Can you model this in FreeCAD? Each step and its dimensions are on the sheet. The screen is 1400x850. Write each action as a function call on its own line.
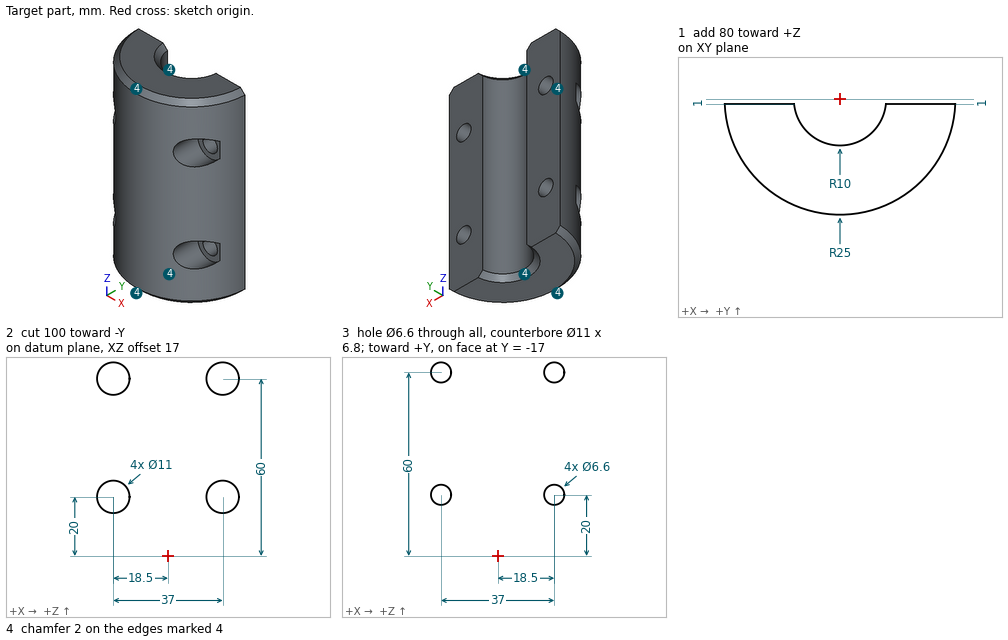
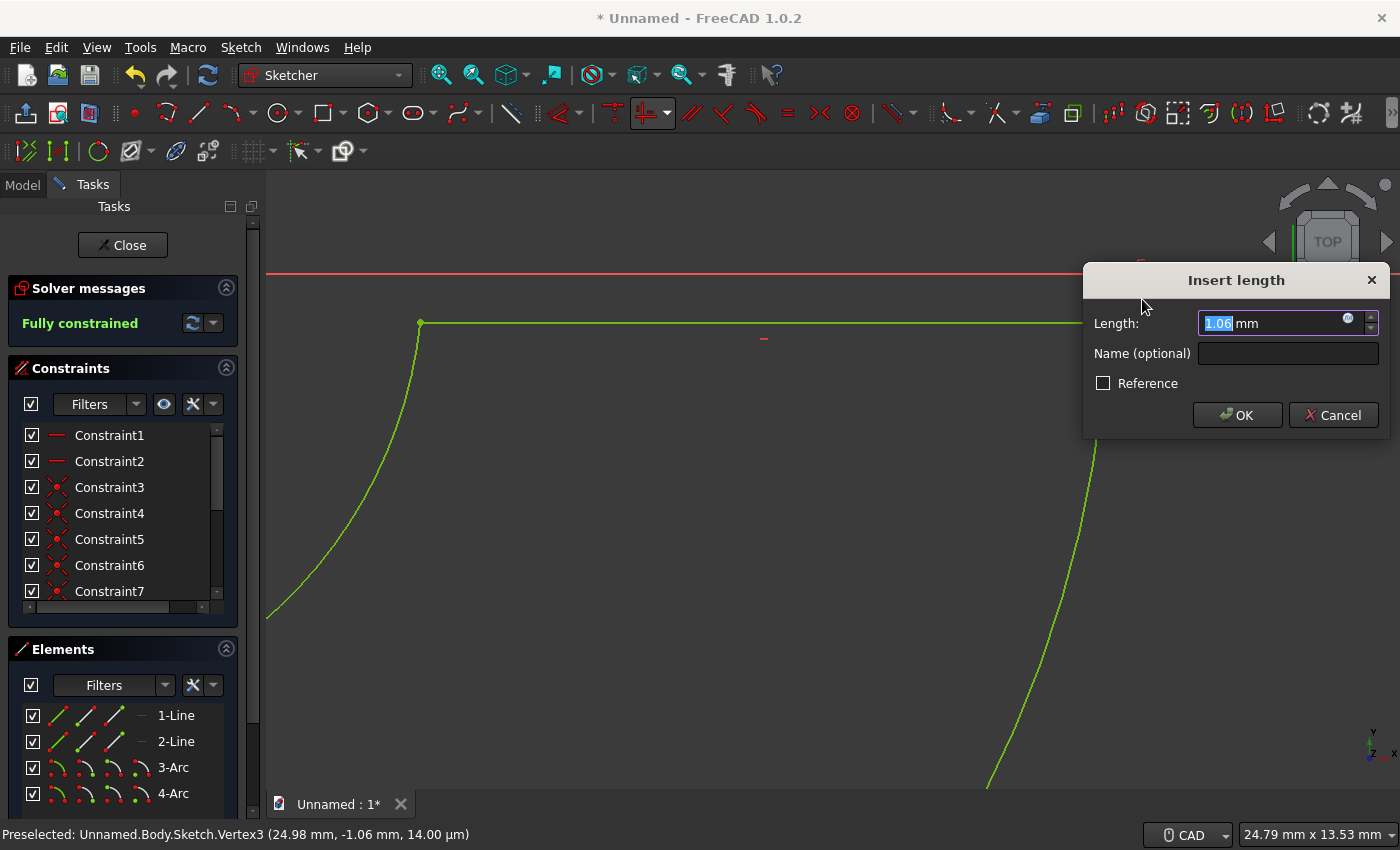
text(1)
key(Return)
key(Escape)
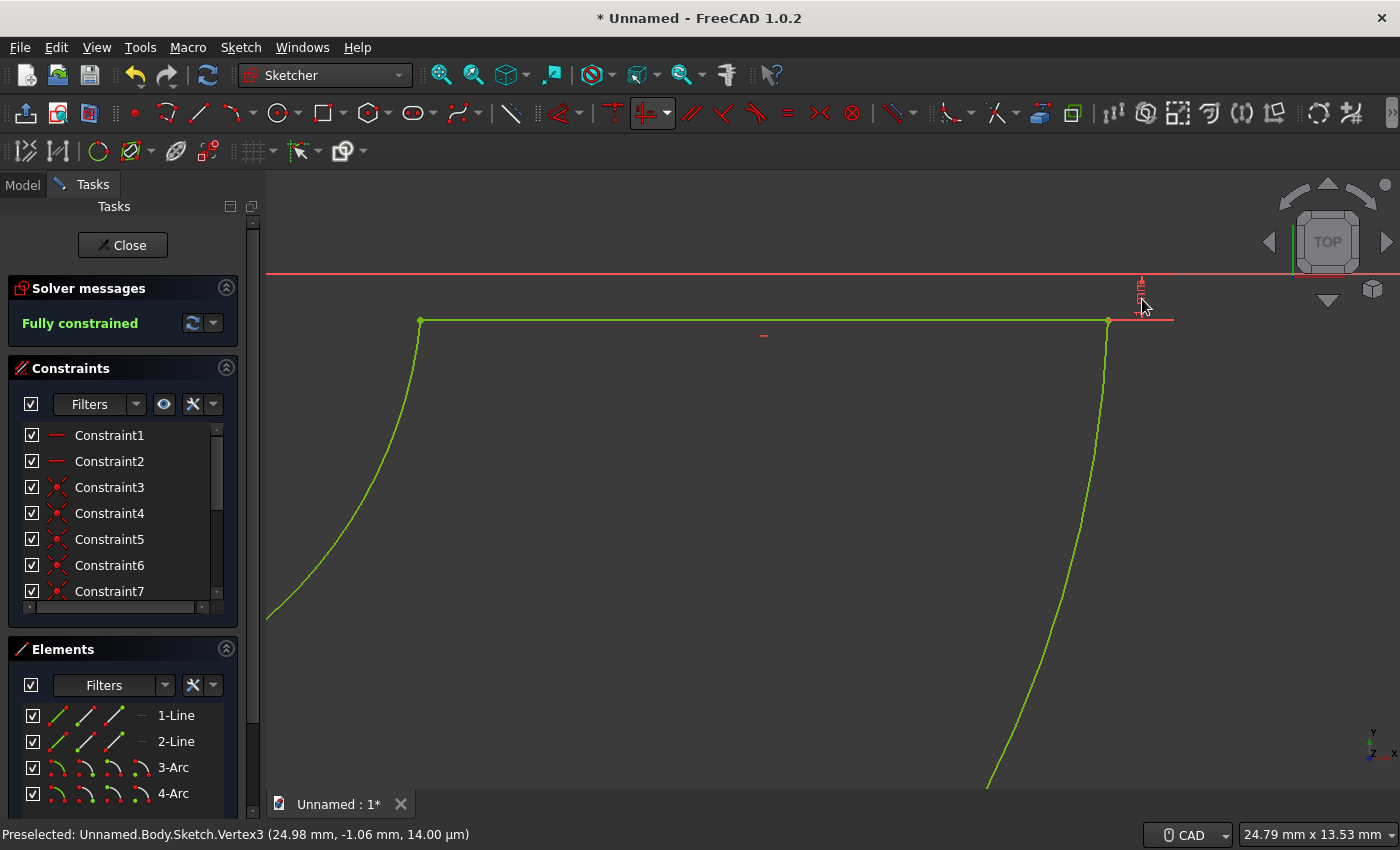
click(123, 245)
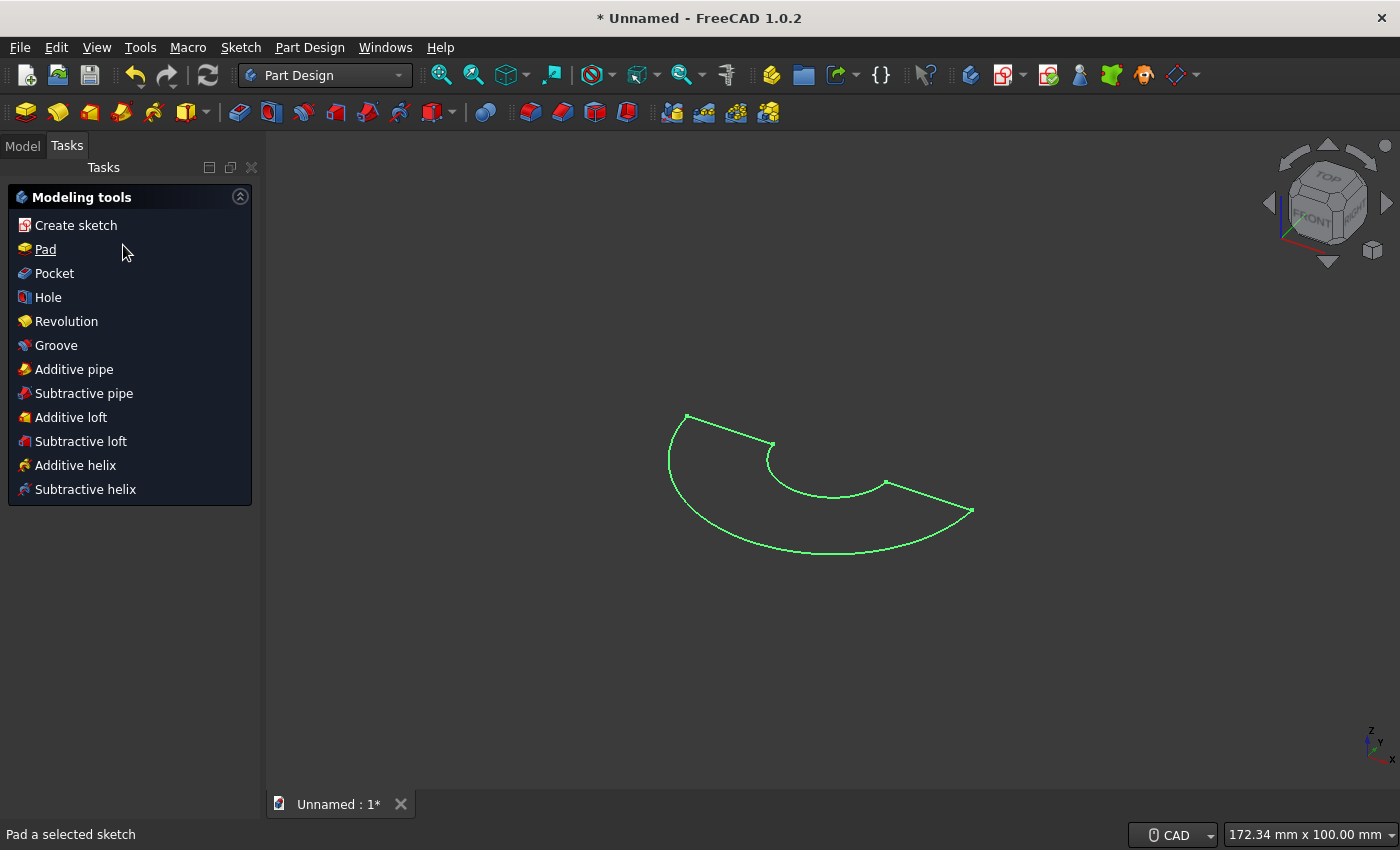
click(26, 112)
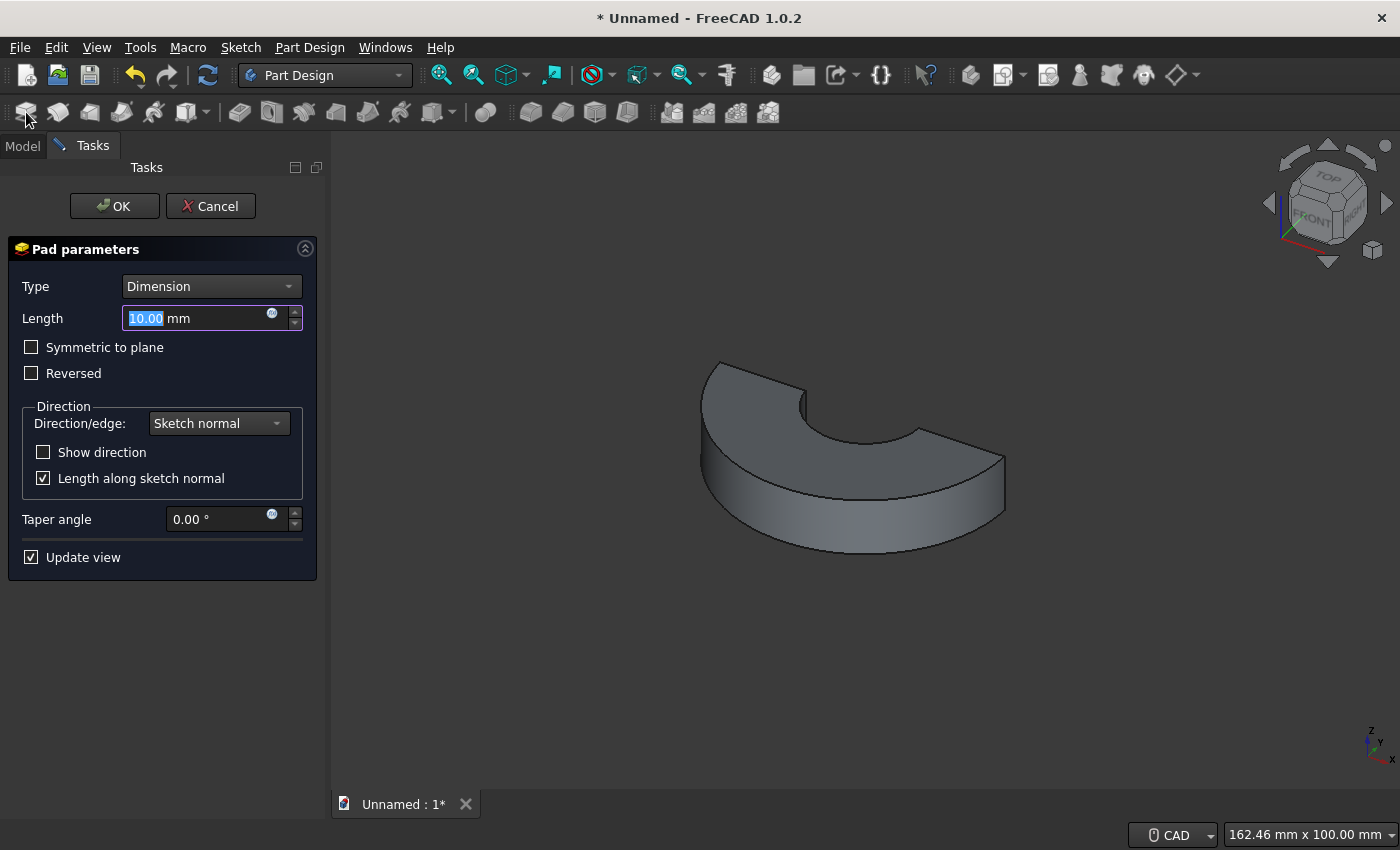
text(80)
key(Tab)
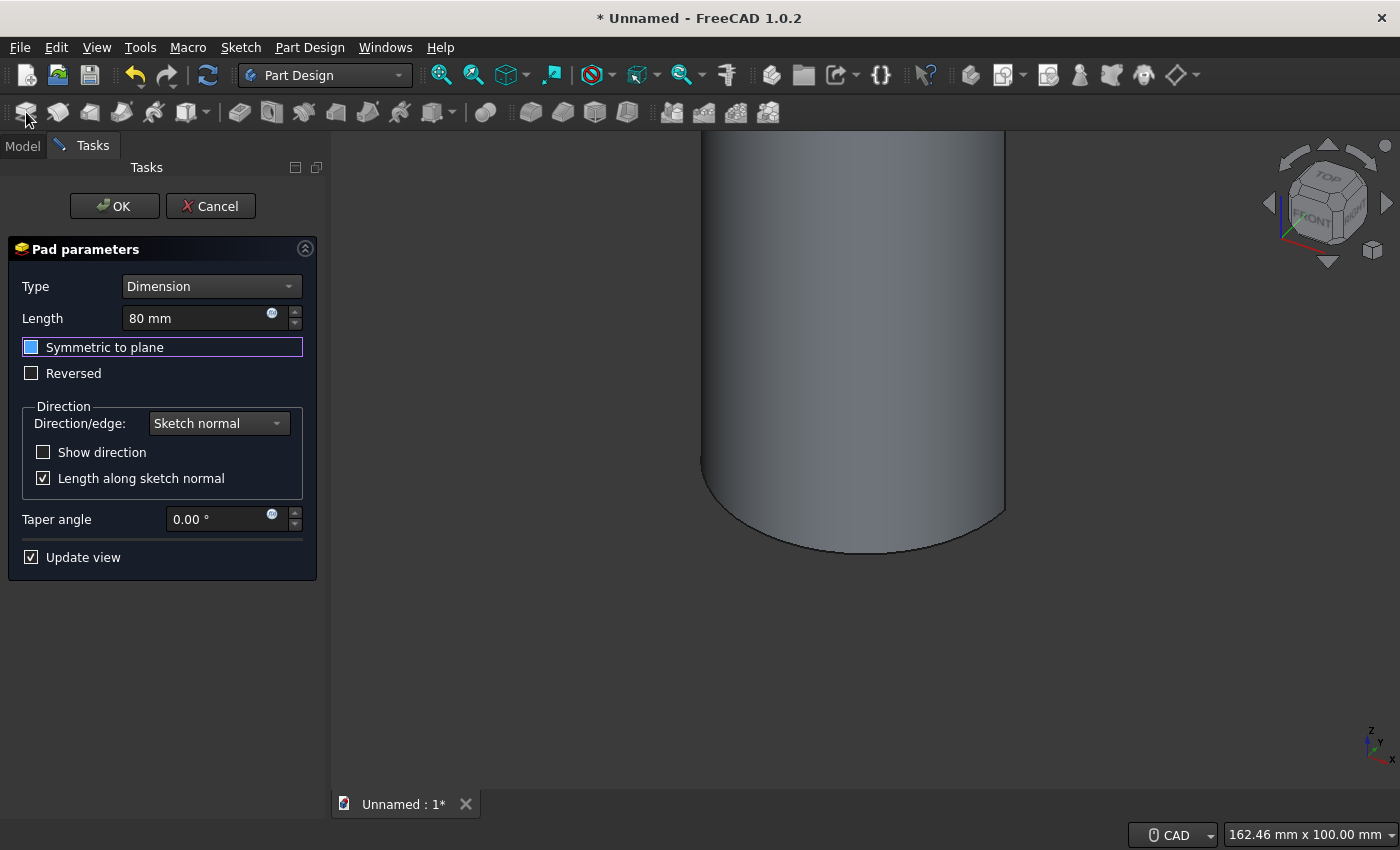
click(115, 206)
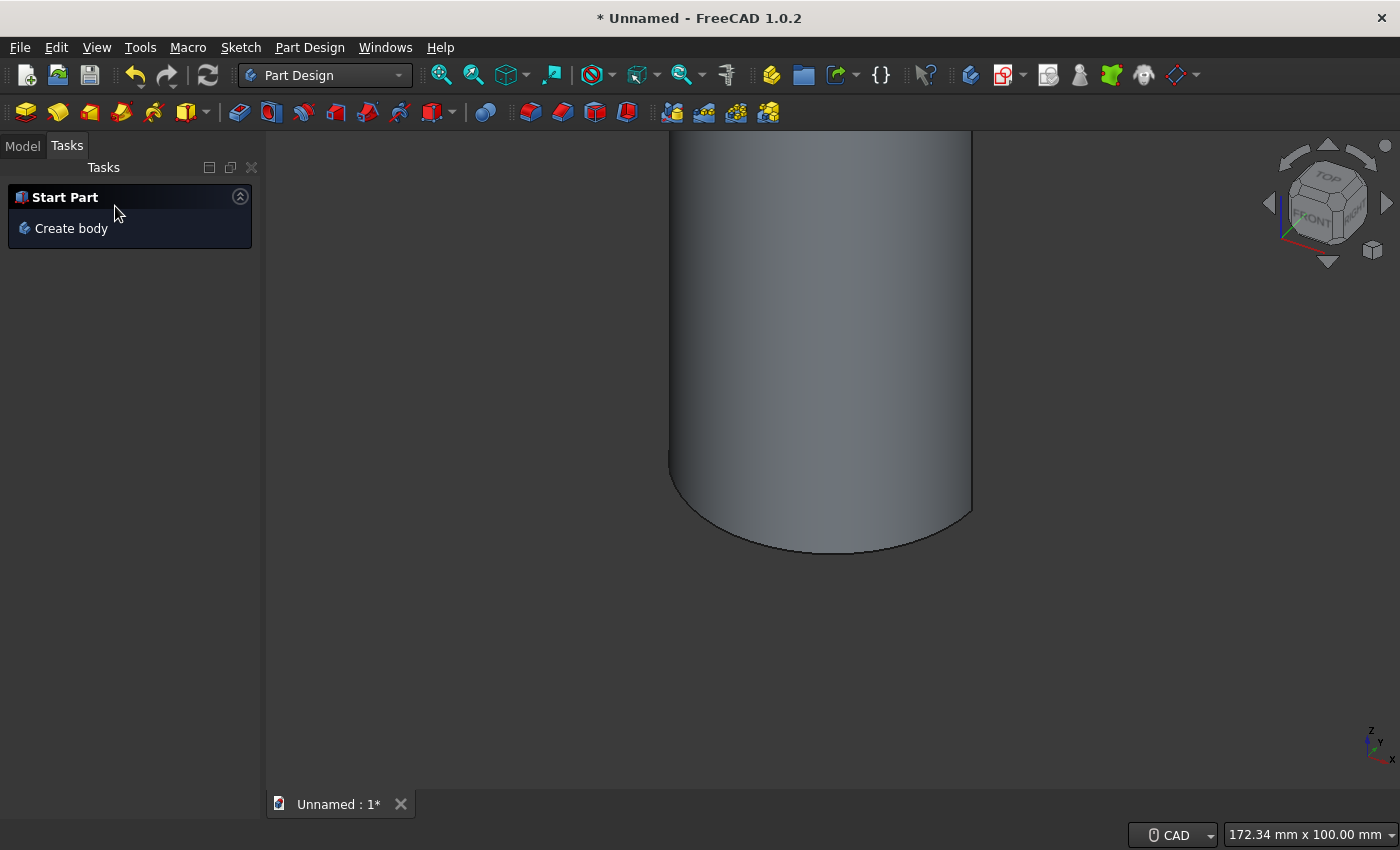
click(442, 76)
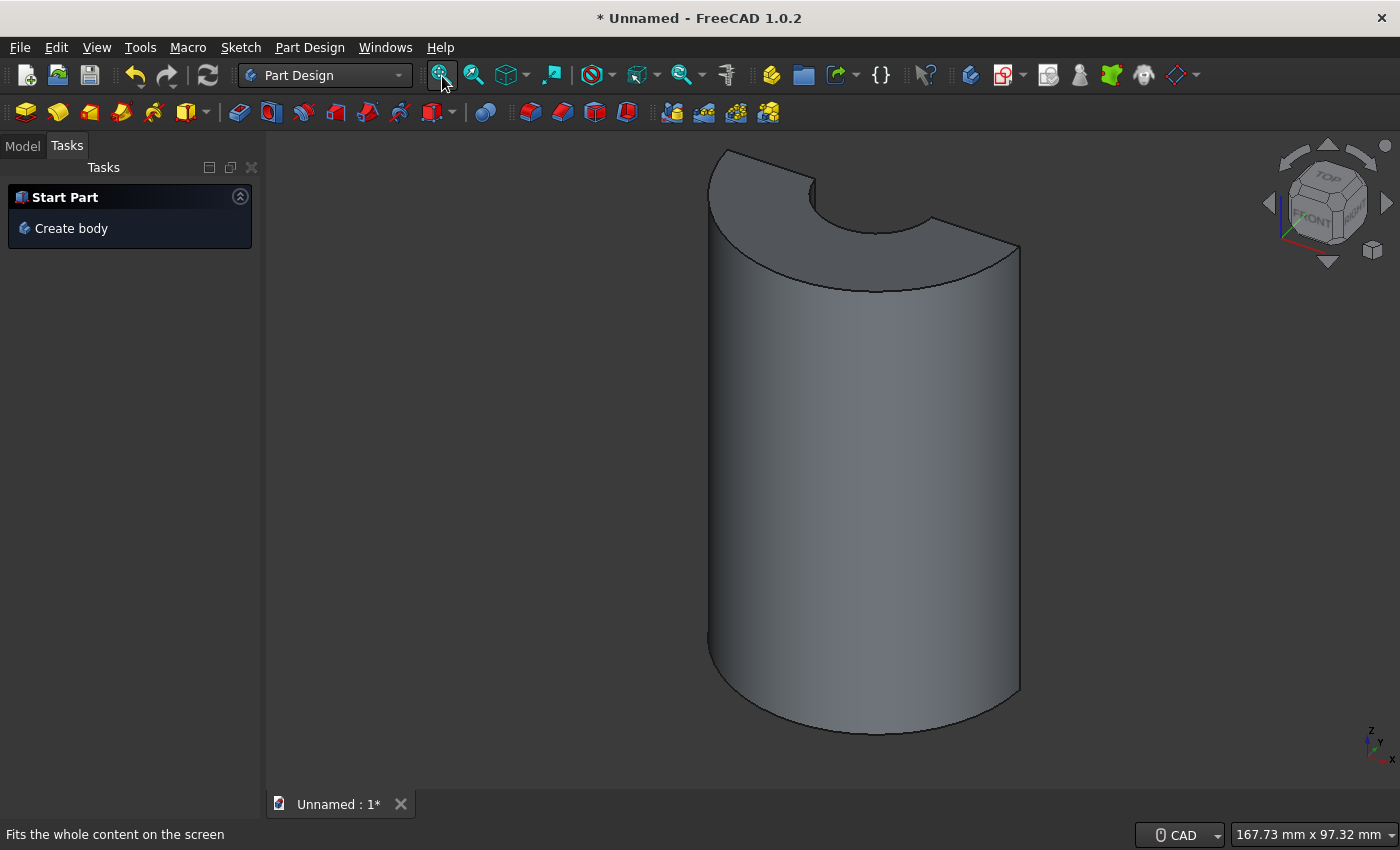
click(23, 145)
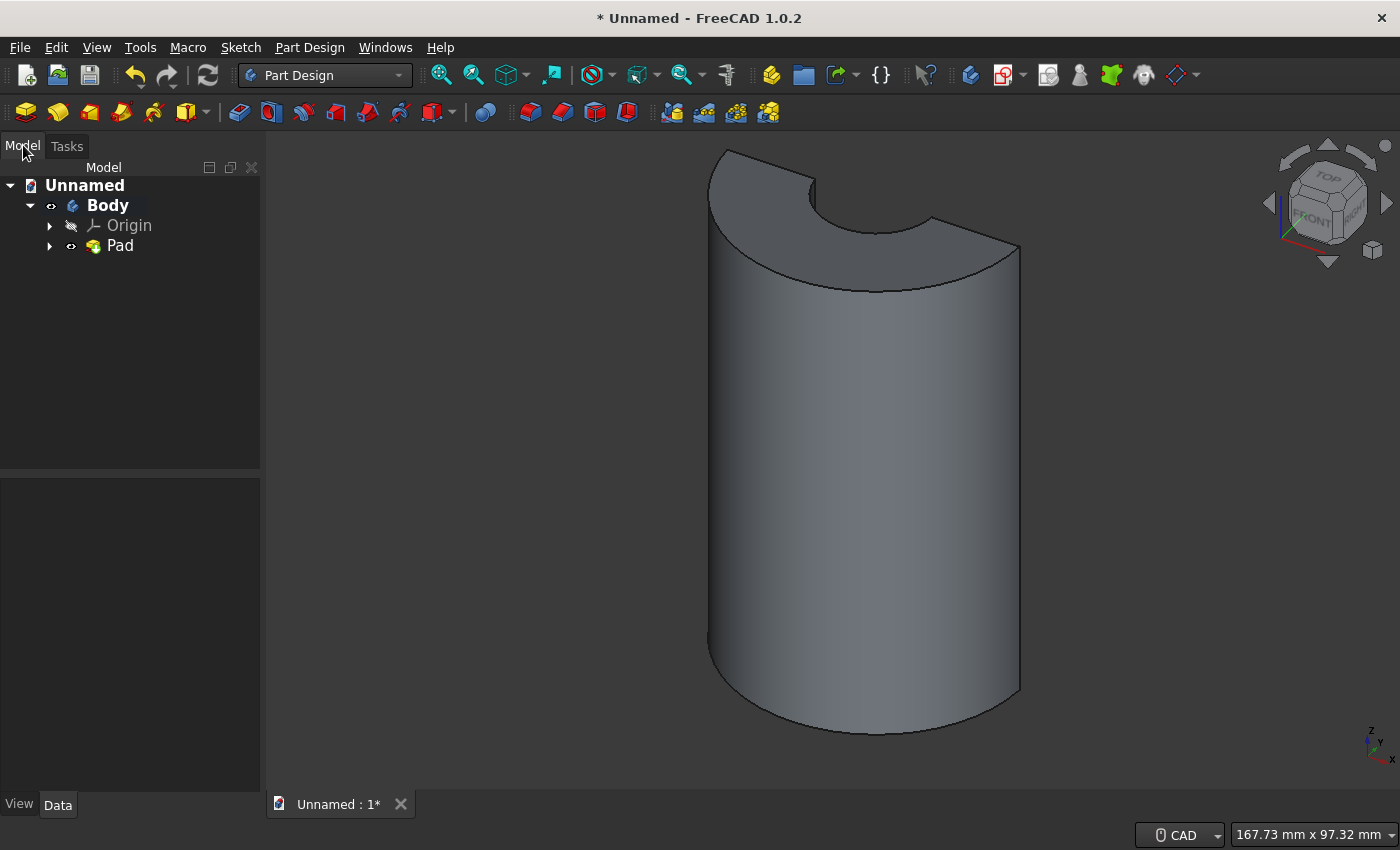
click(50, 226)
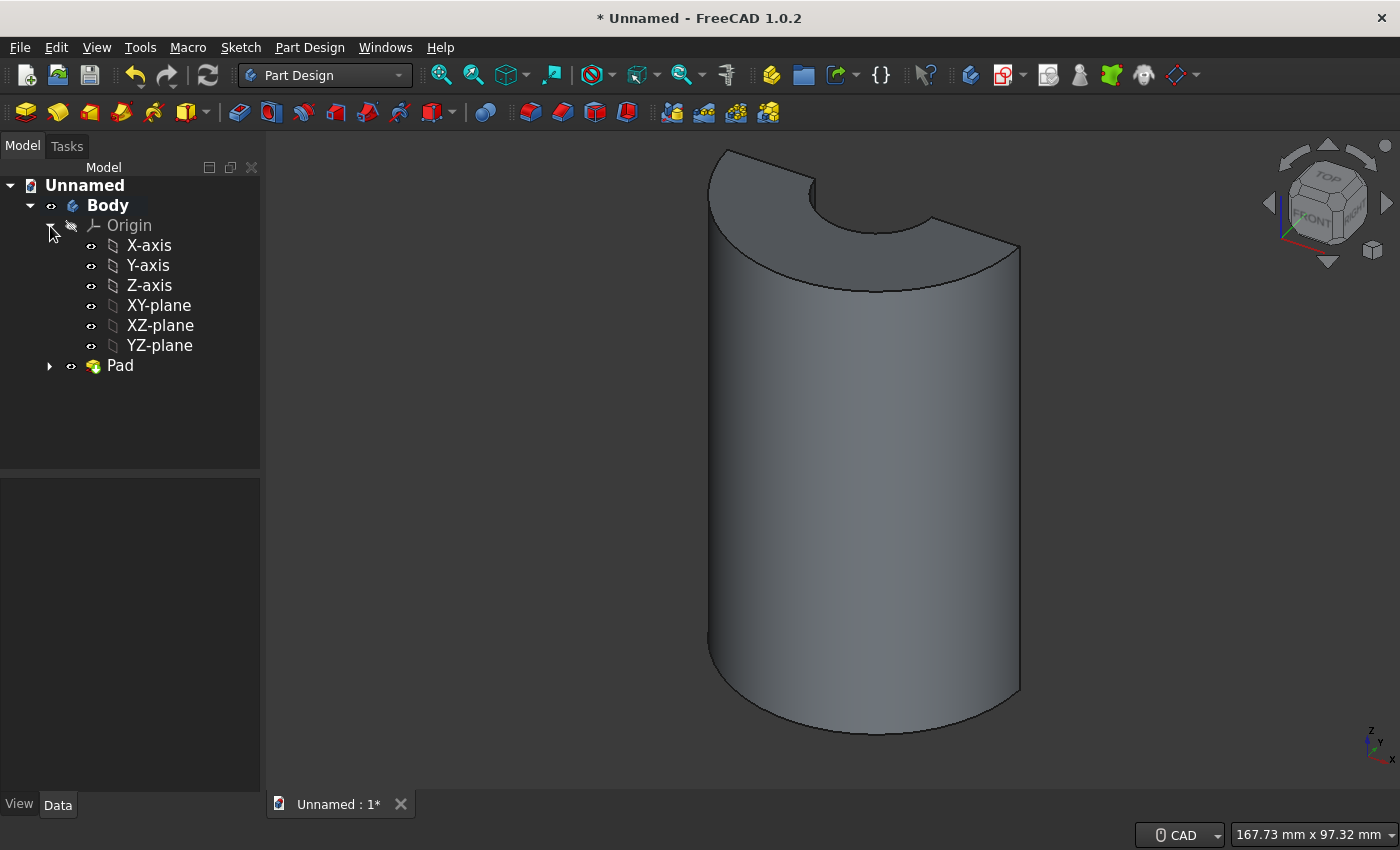
click(136, 326)